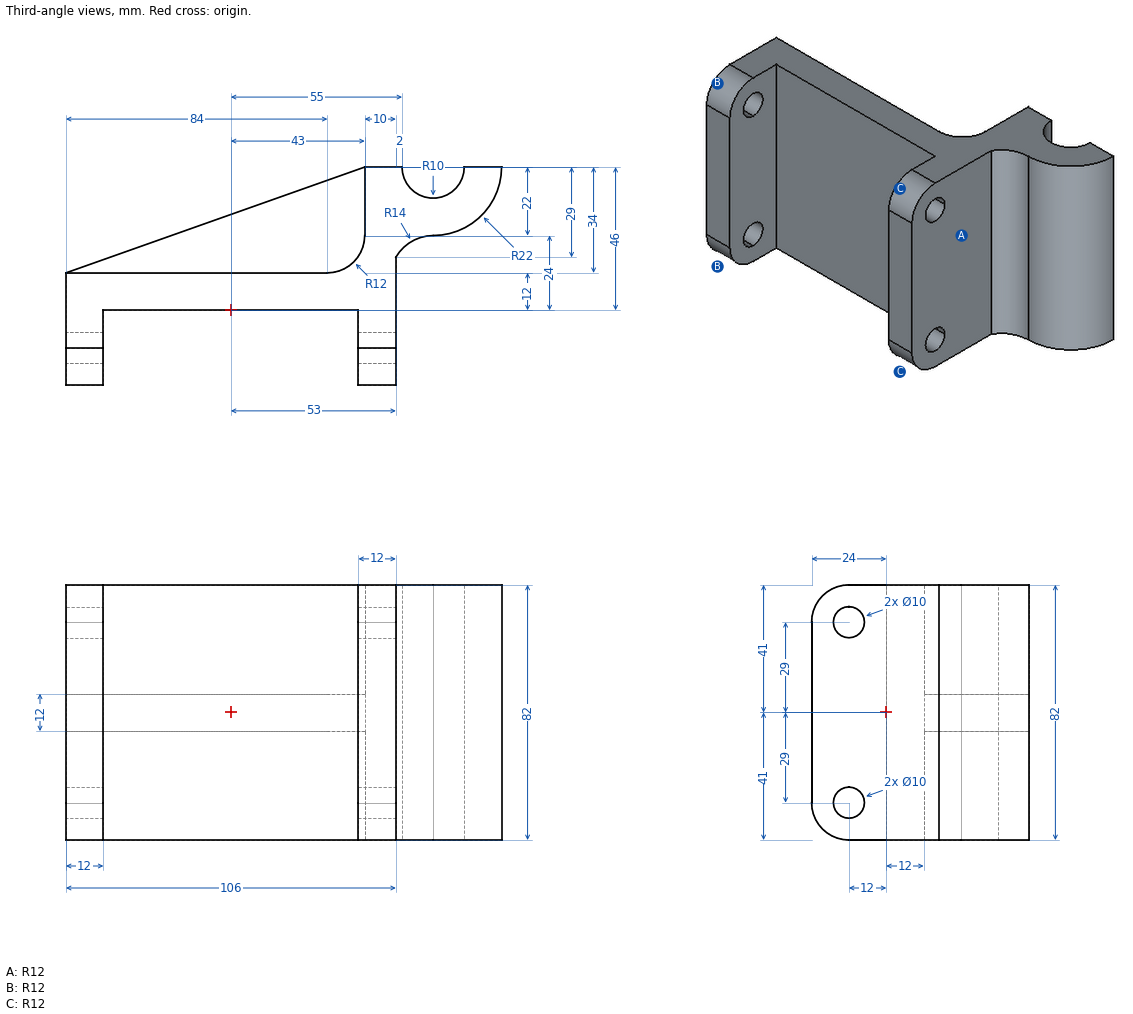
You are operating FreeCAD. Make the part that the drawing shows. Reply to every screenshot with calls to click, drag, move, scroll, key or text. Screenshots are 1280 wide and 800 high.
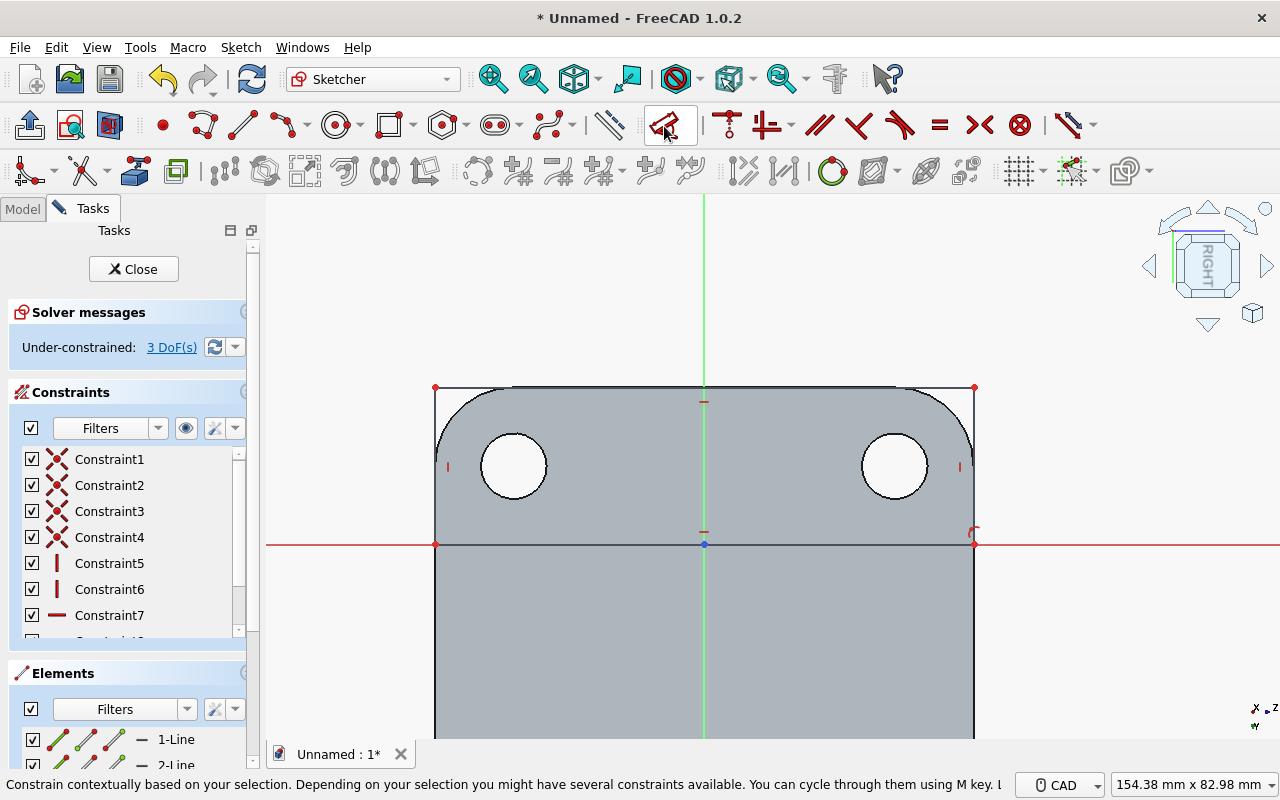
click(435, 435)
click(401, 466)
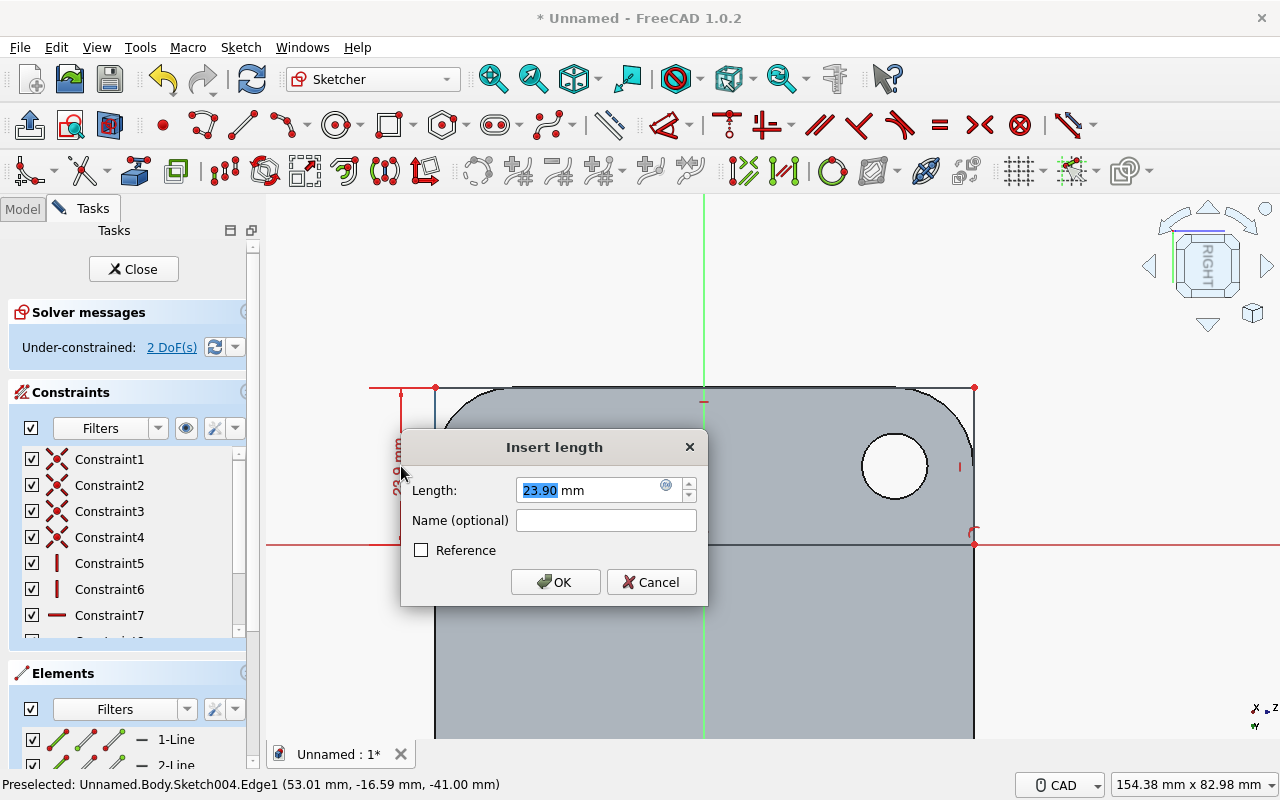
text(24)
key(Return)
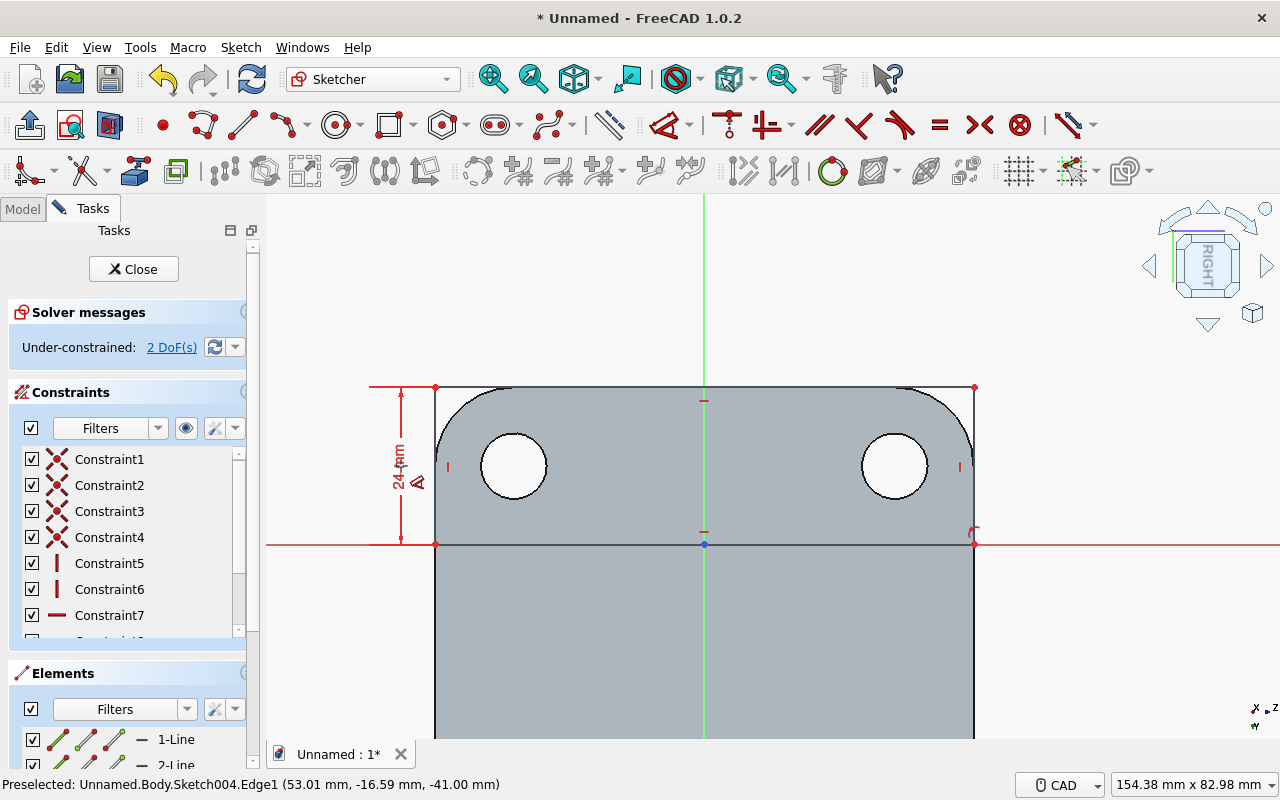
click(597, 545)
click(581, 579)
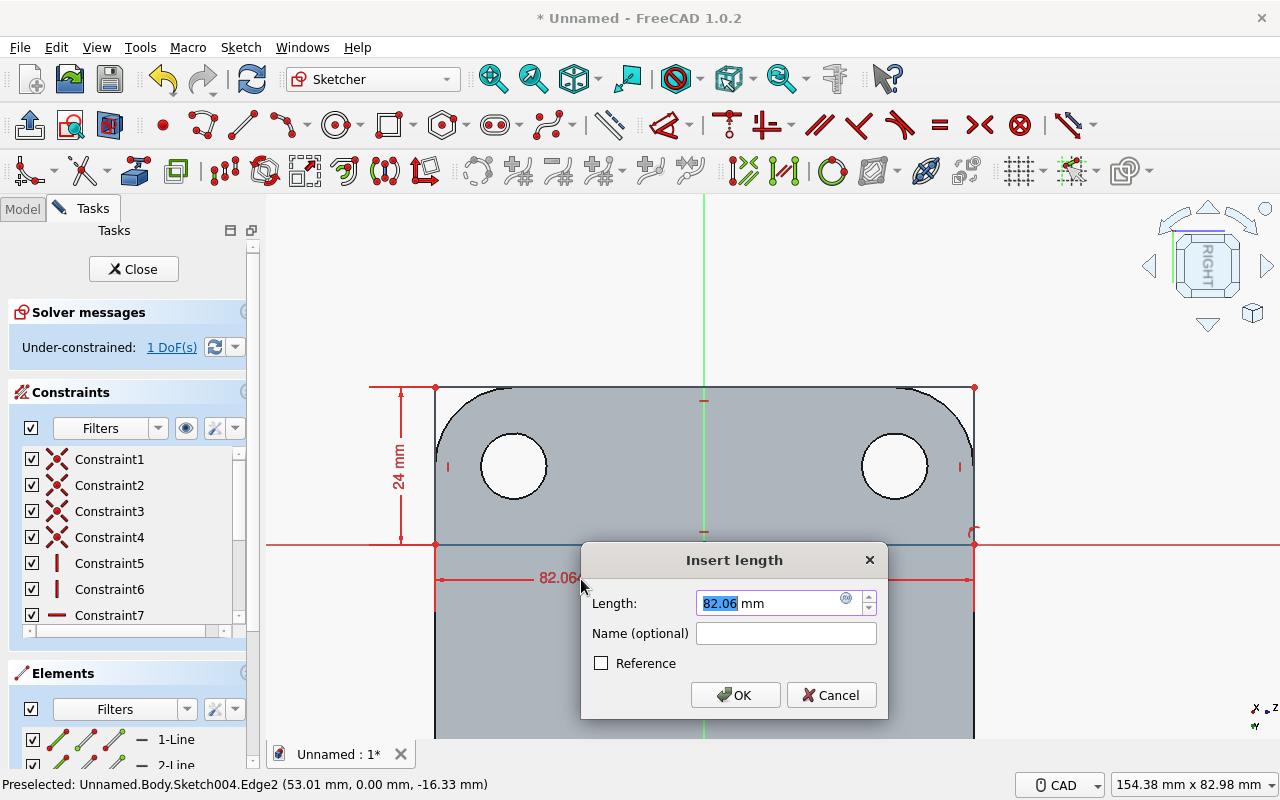
text(82)
key(Return)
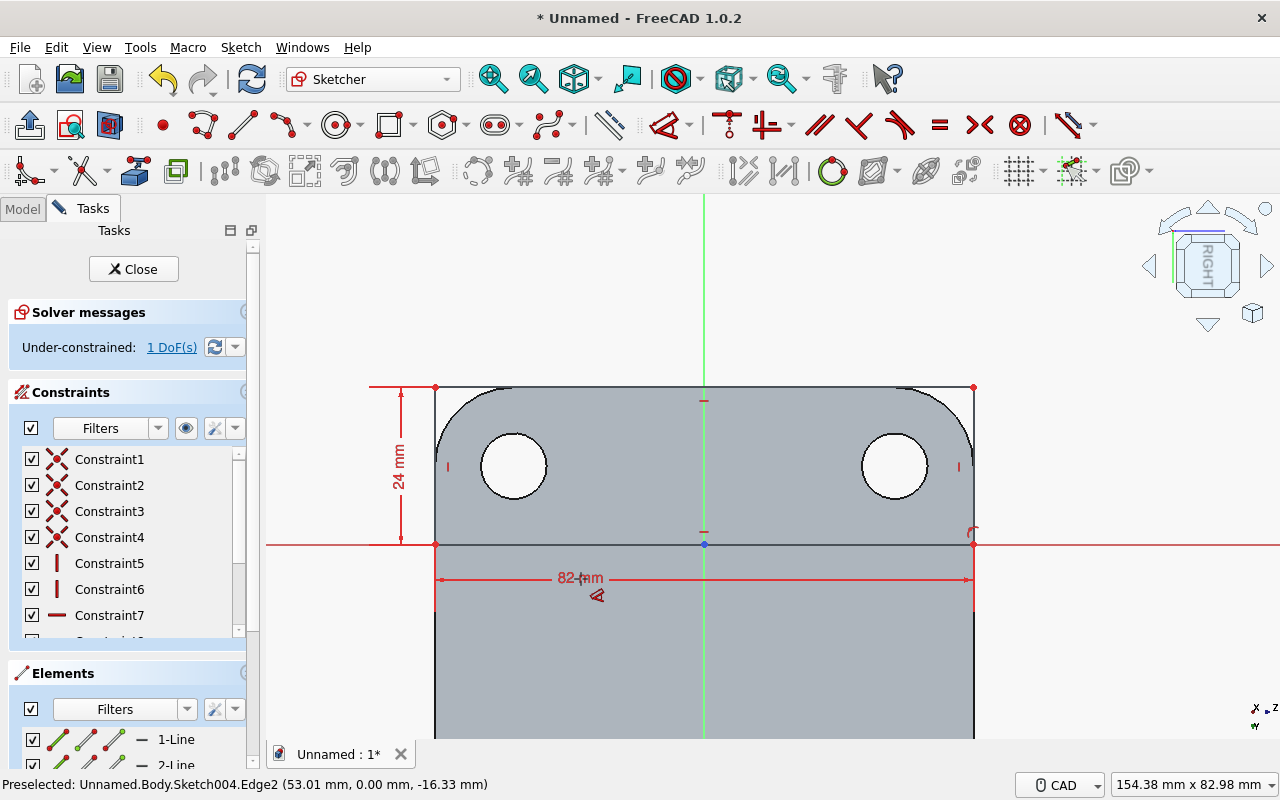
click(435, 387)
click(508, 579)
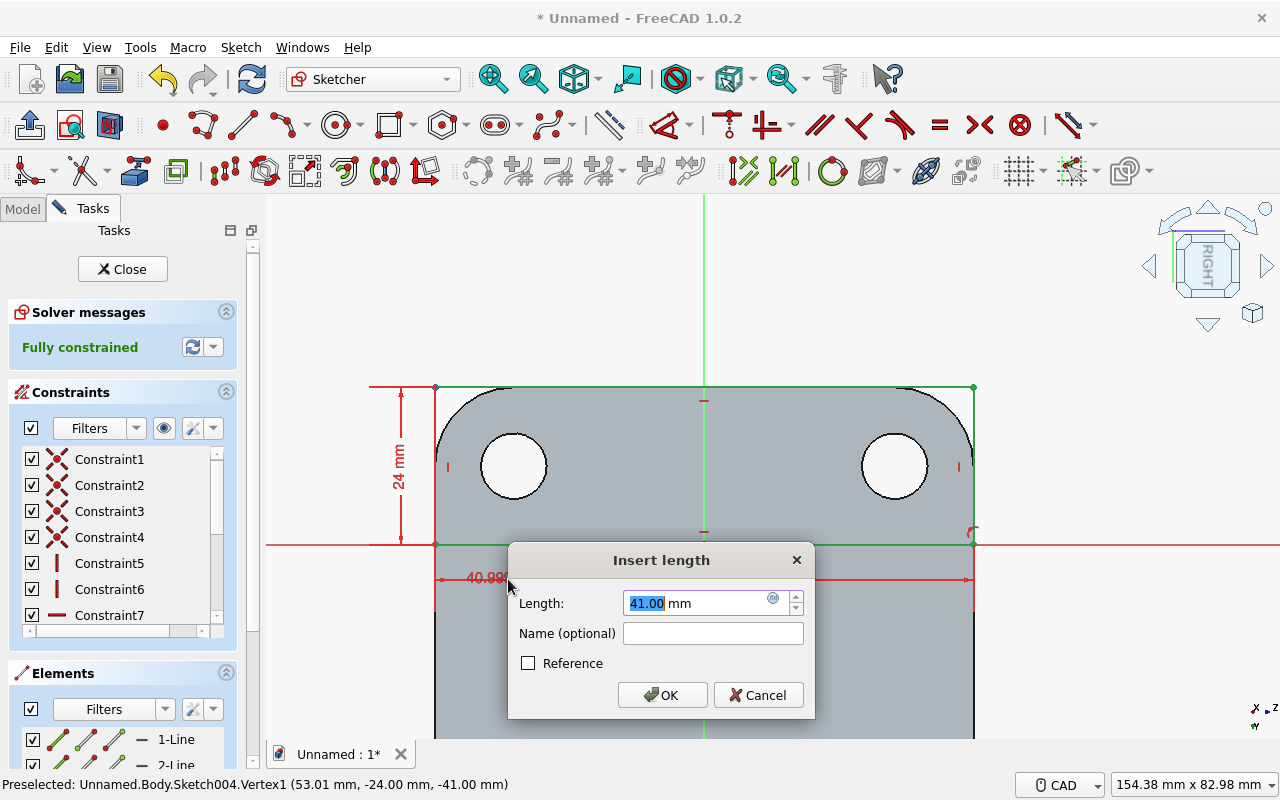
text(41)
key(Return)
key(Escape)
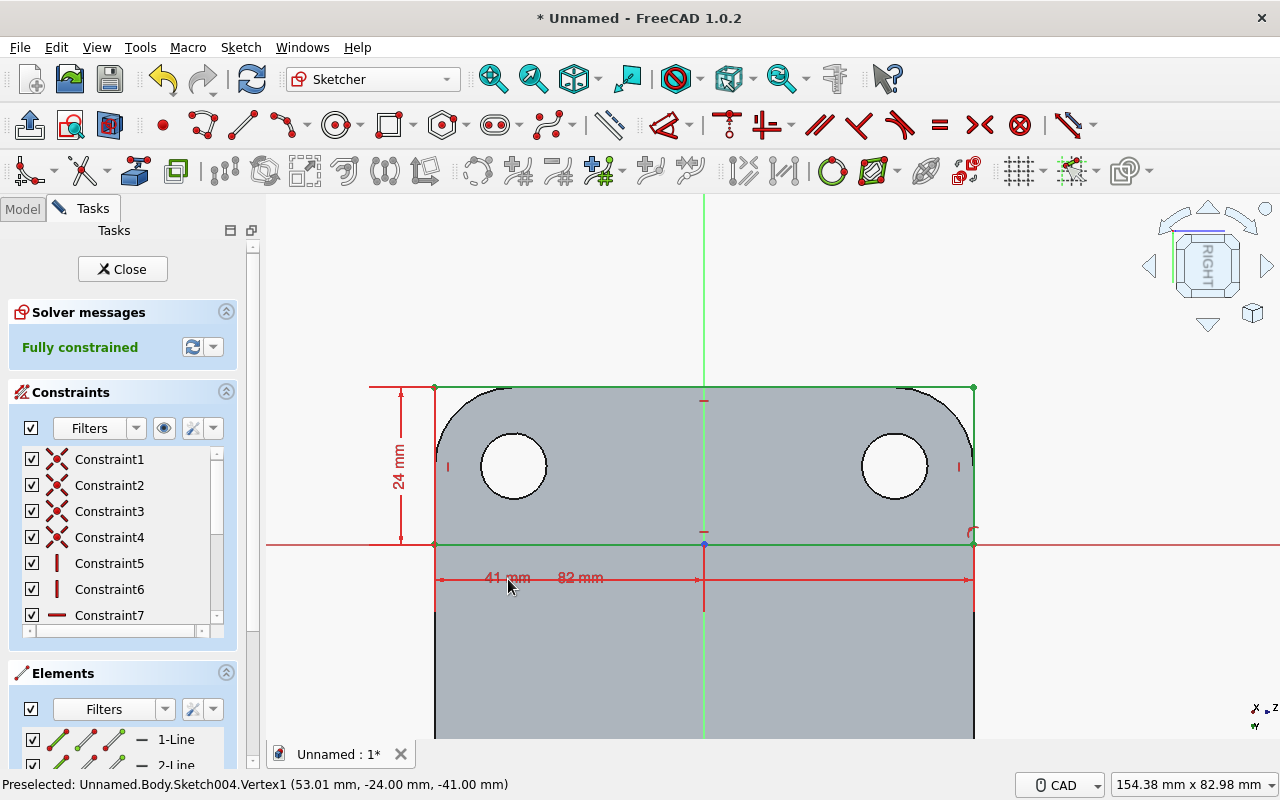
click(123, 269)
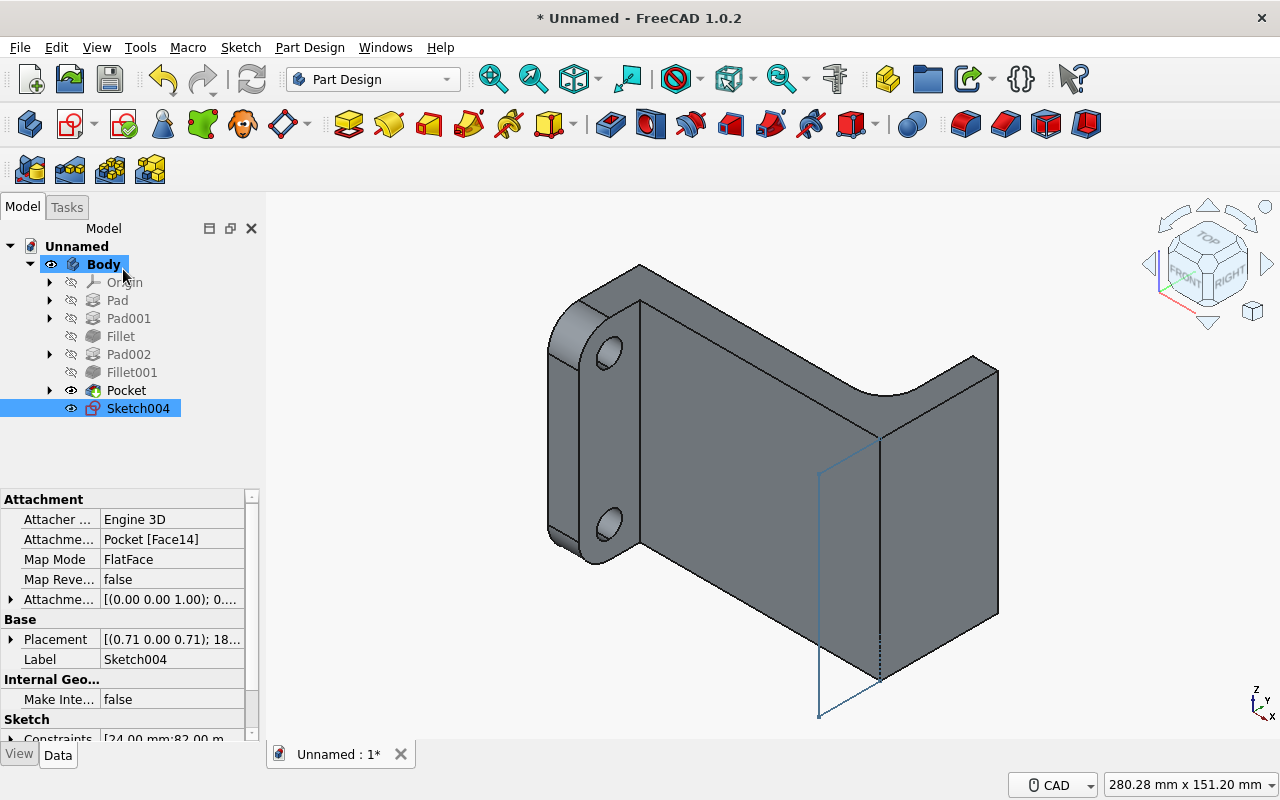
click(350, 124)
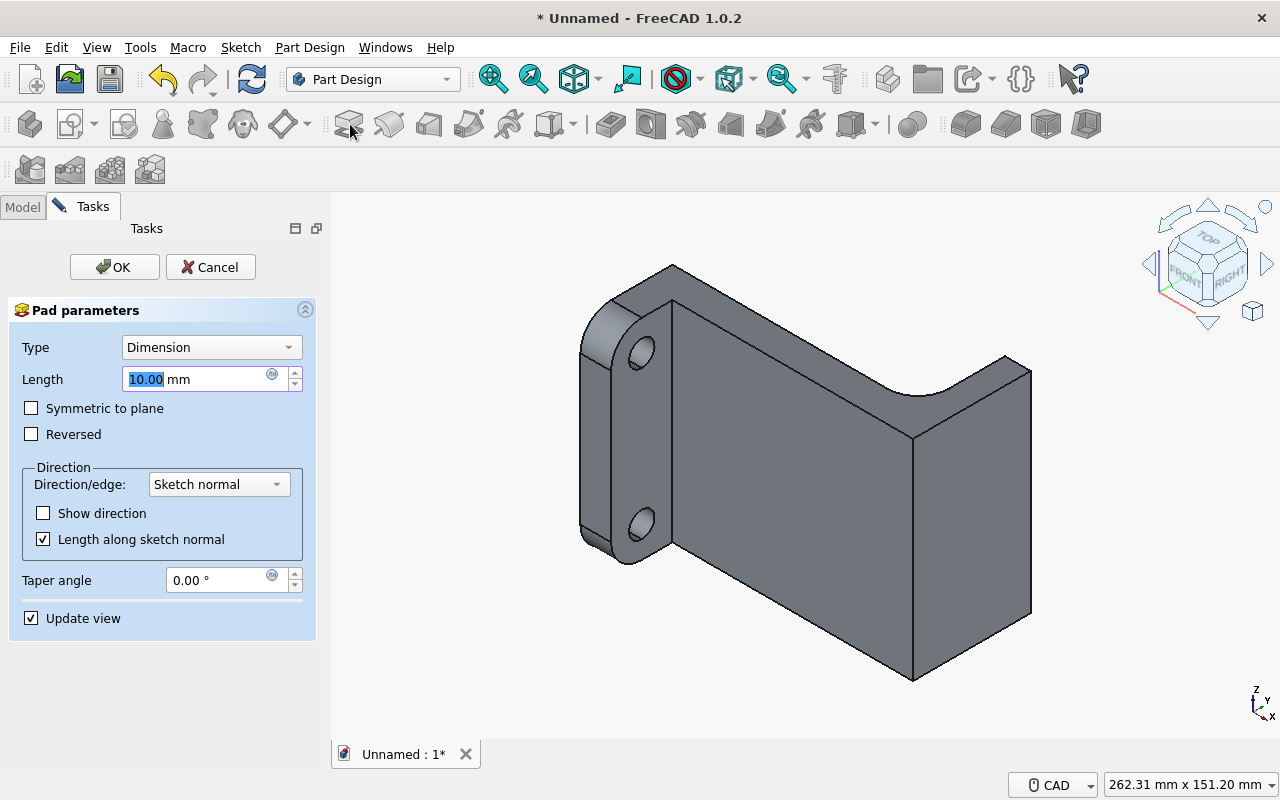
text(12)
key(Tab)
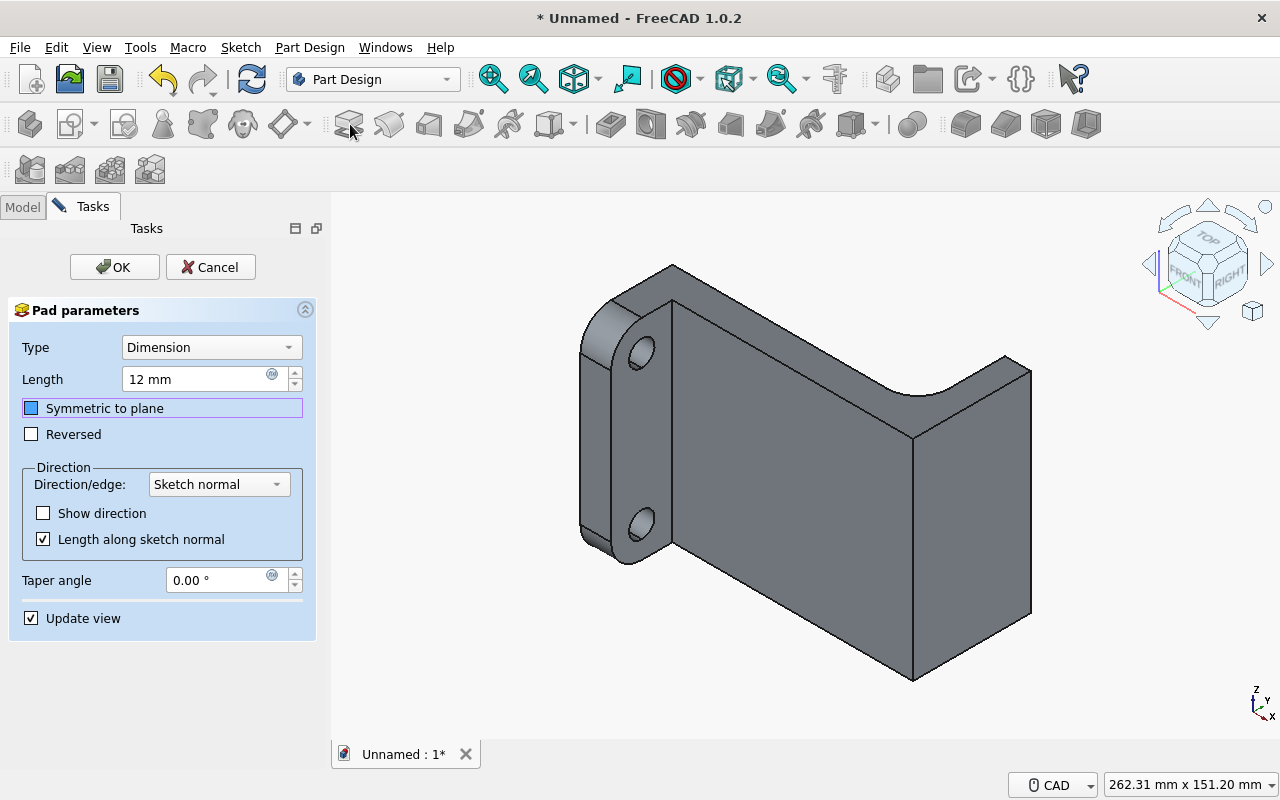
click(30, 434)